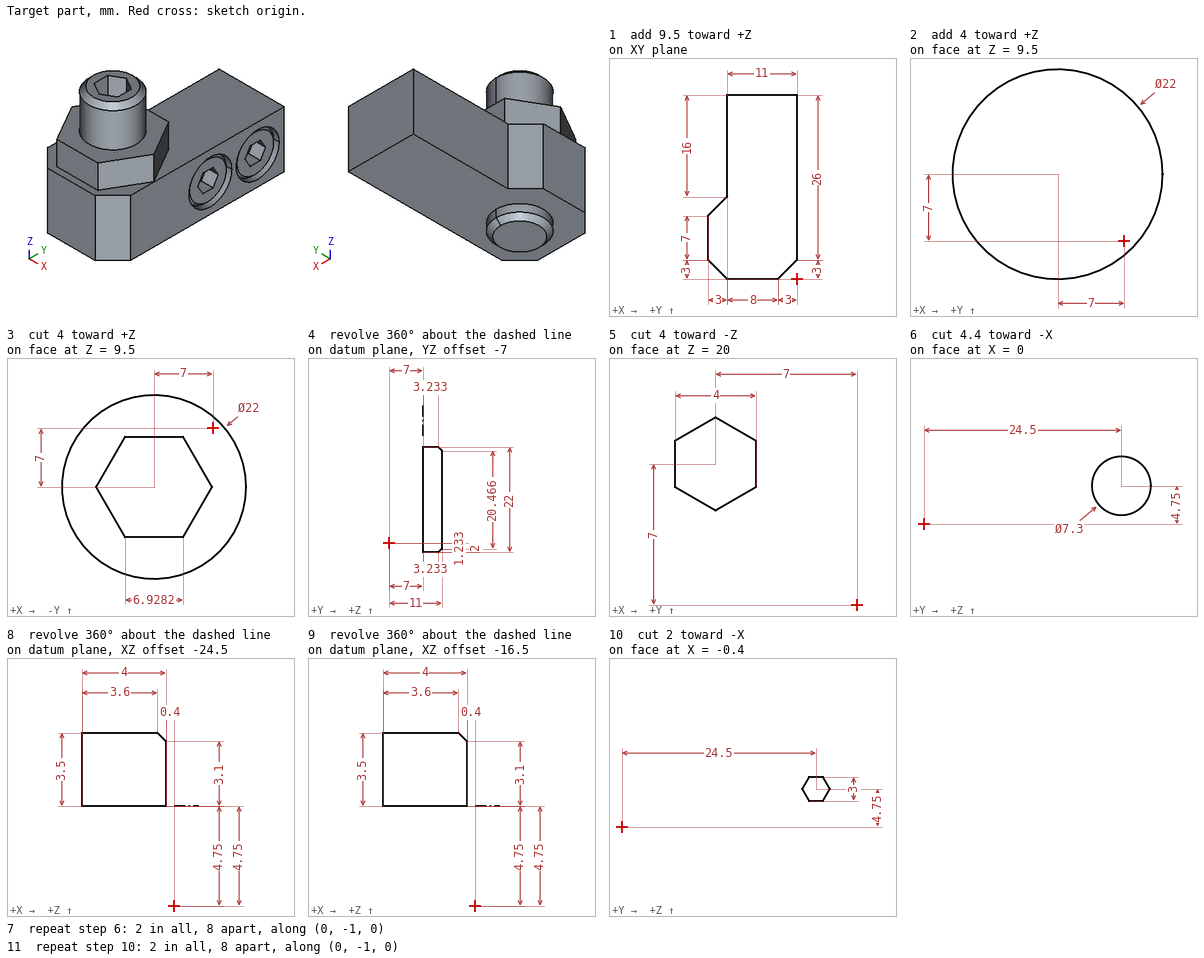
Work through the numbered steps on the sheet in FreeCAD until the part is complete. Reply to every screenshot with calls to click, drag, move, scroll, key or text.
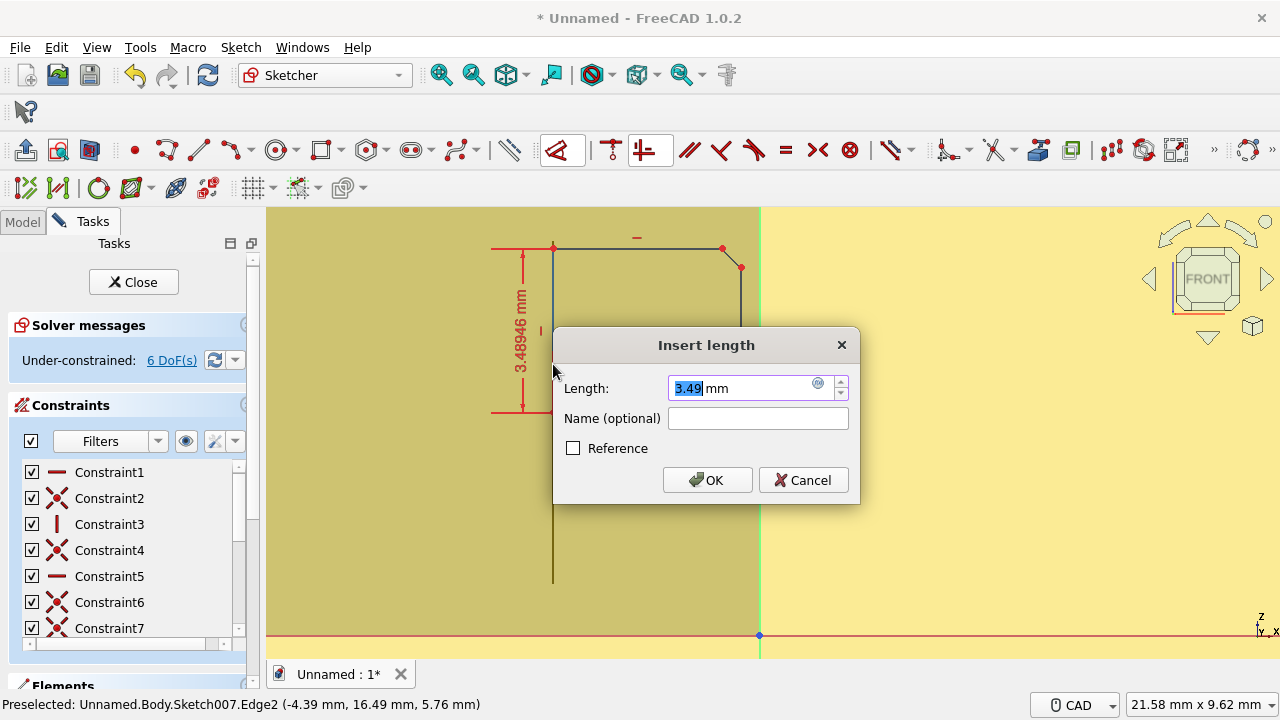
text(3.5)
key(Return)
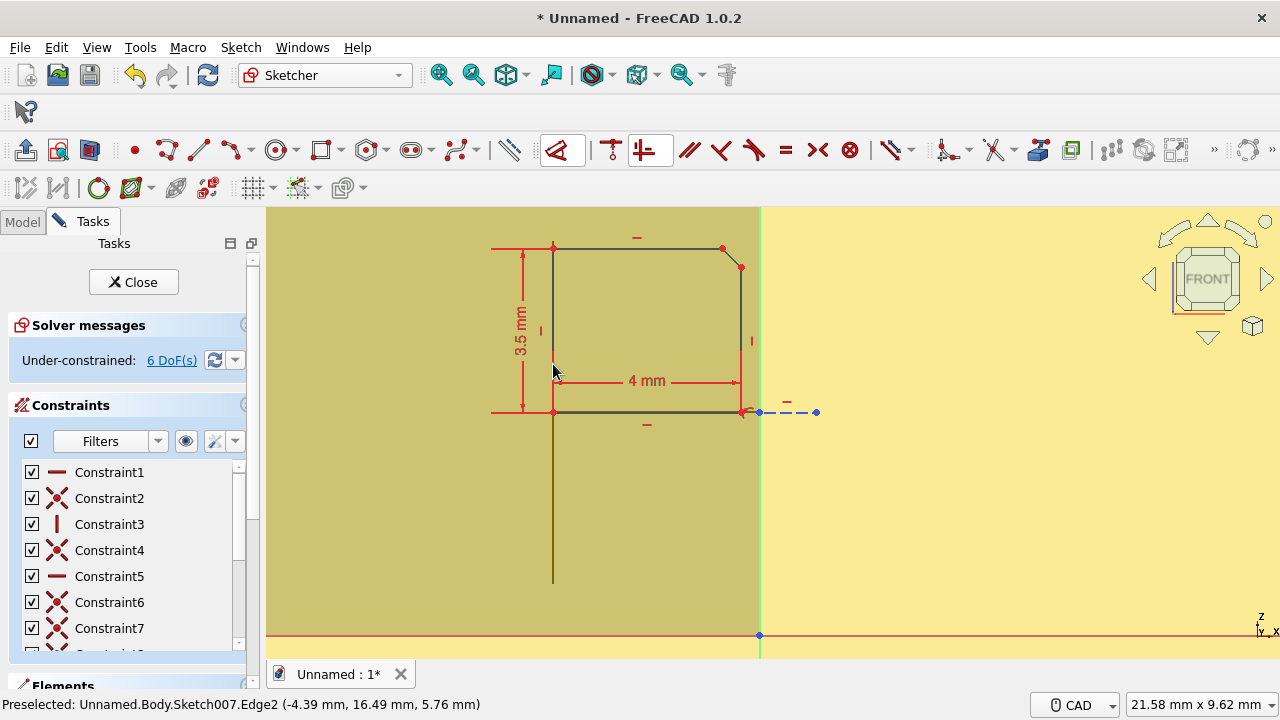
click(604, 249)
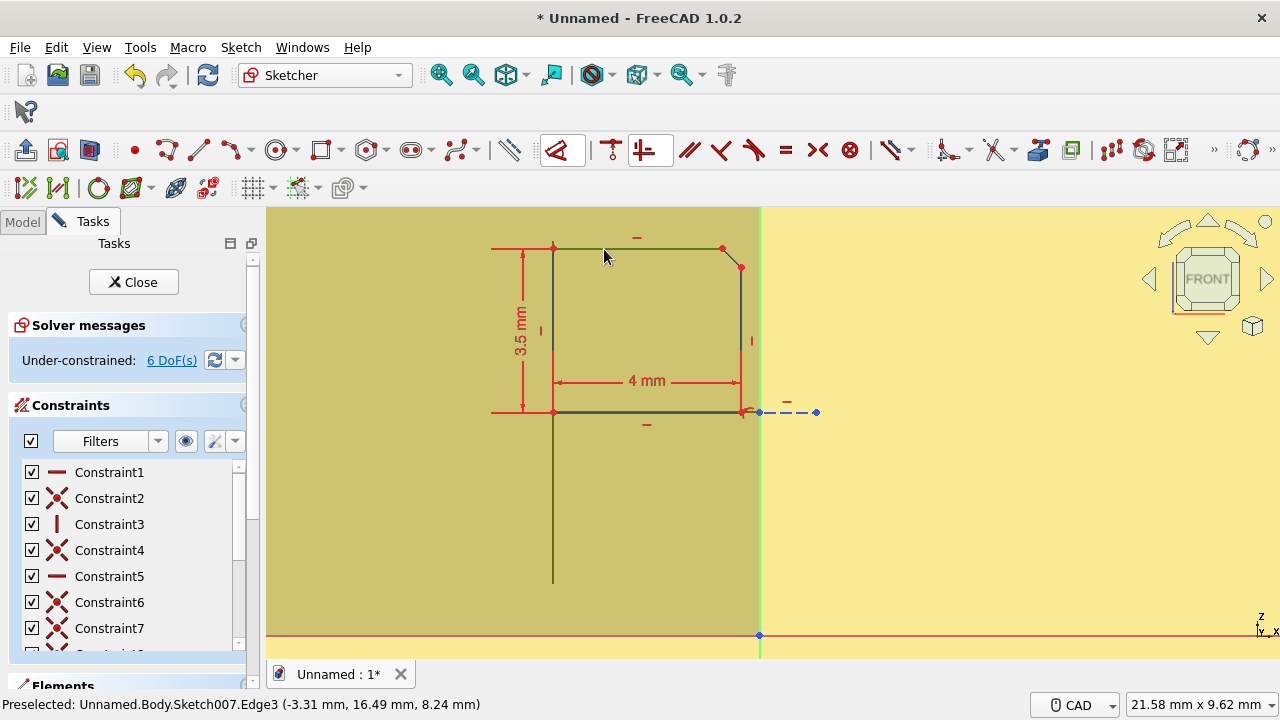
key(l)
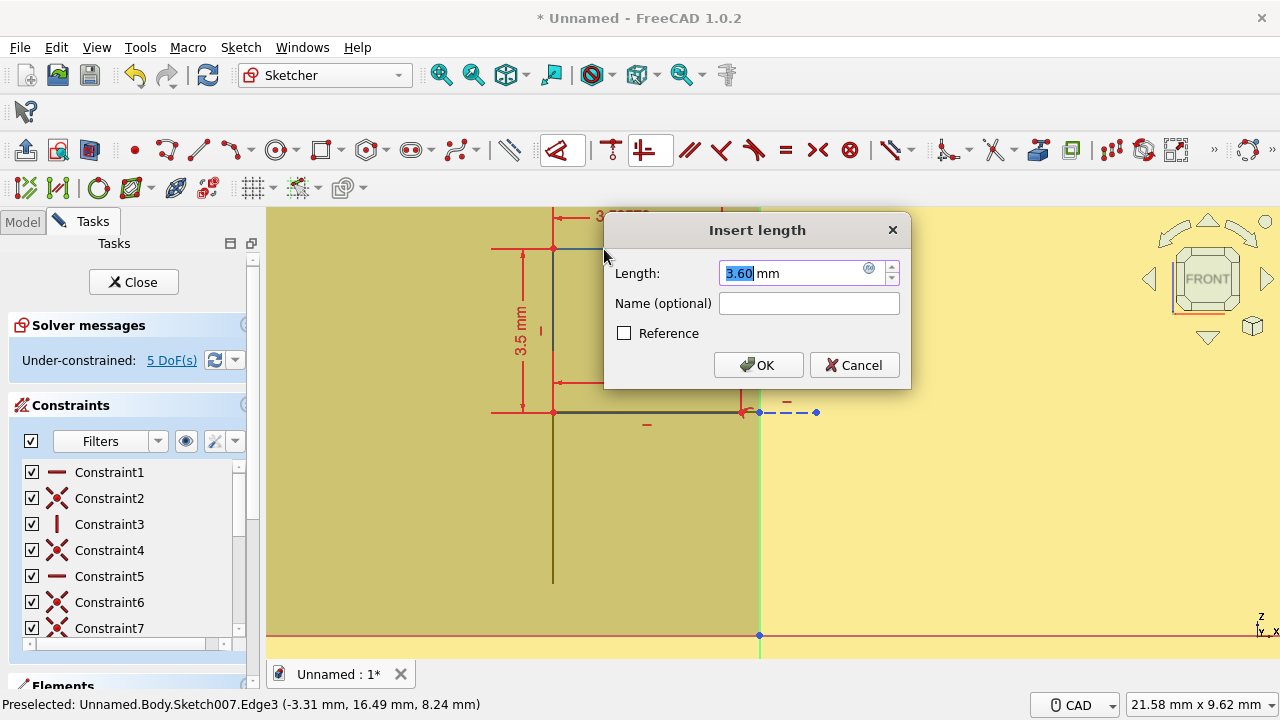
text(3.6)
key(Return)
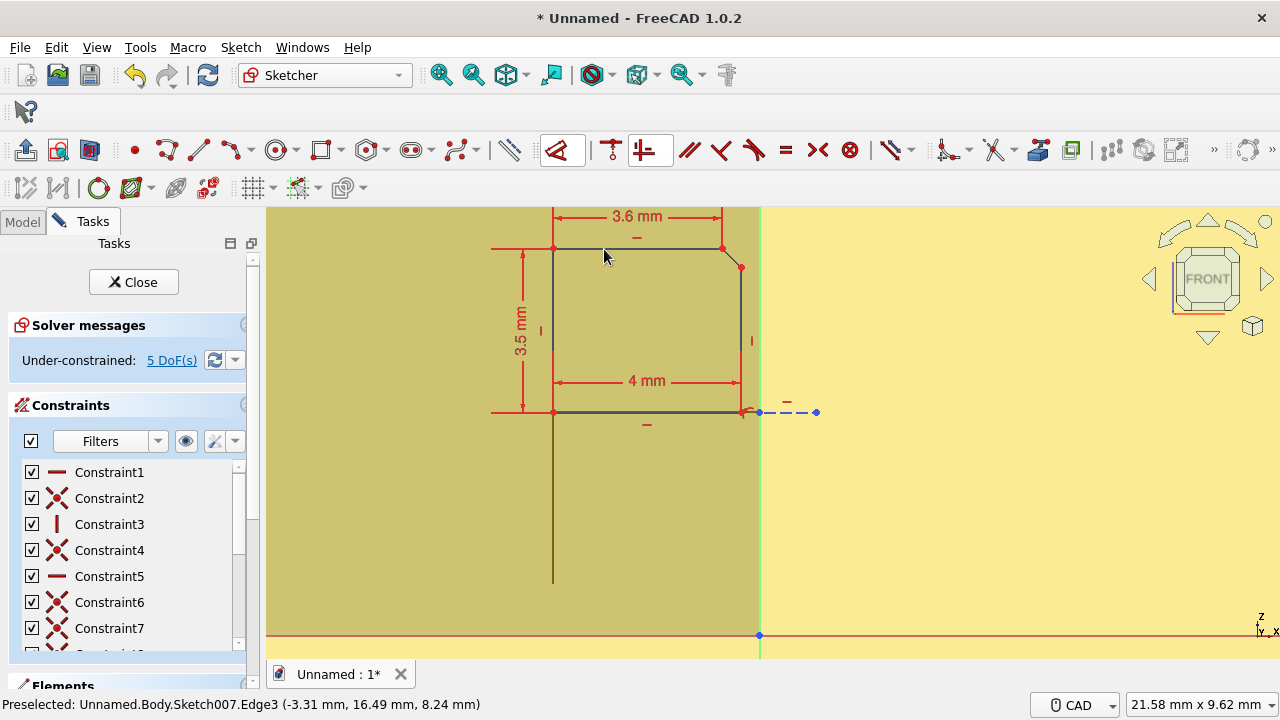
click(741, 312)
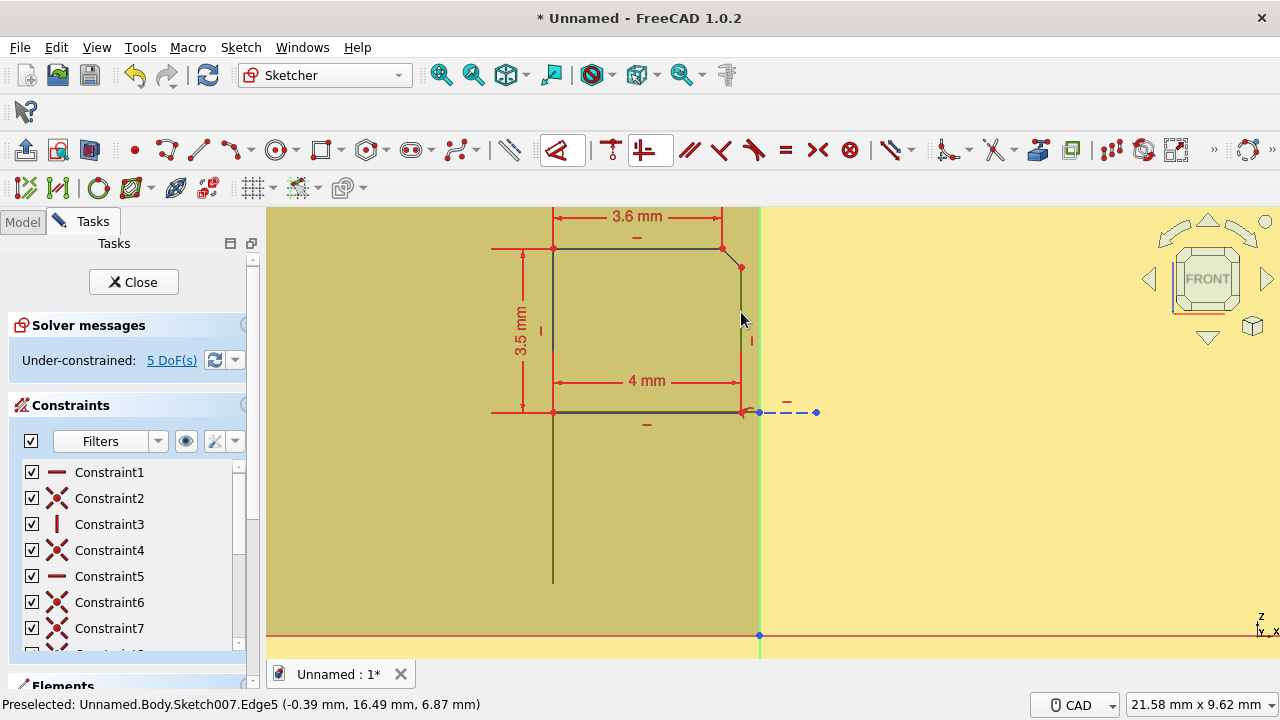
click(580, 150)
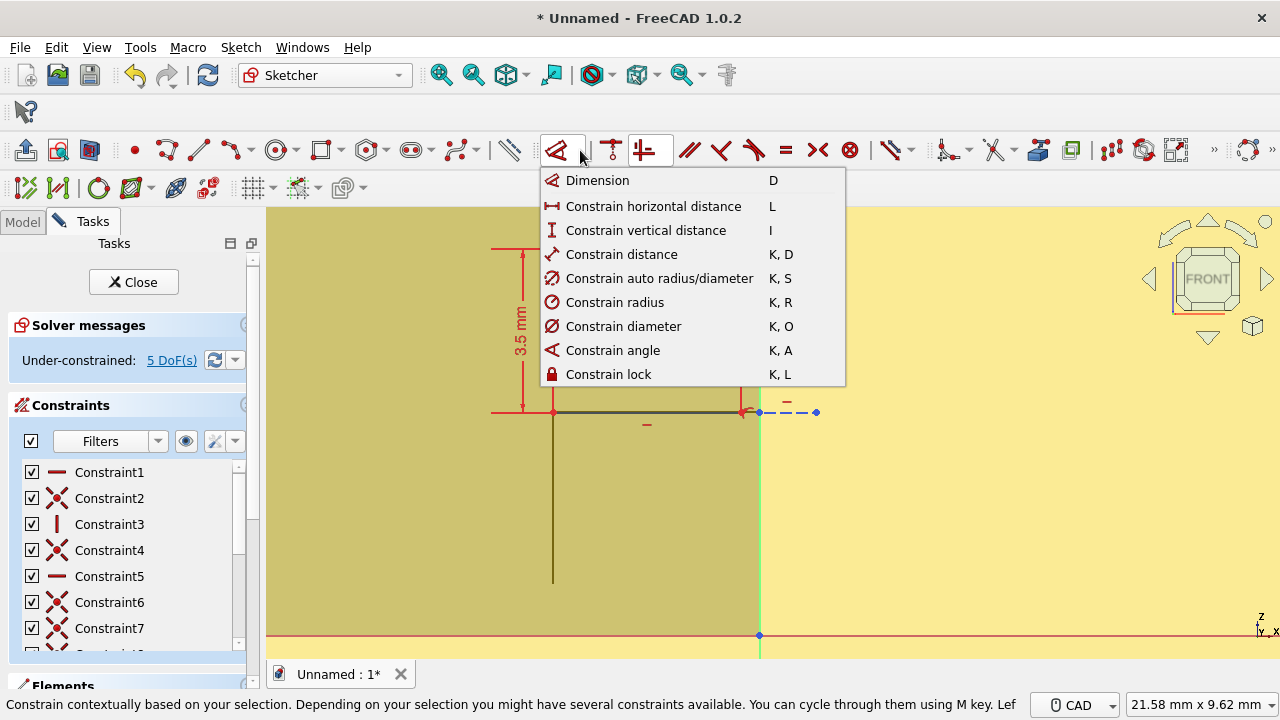
click(693, 230)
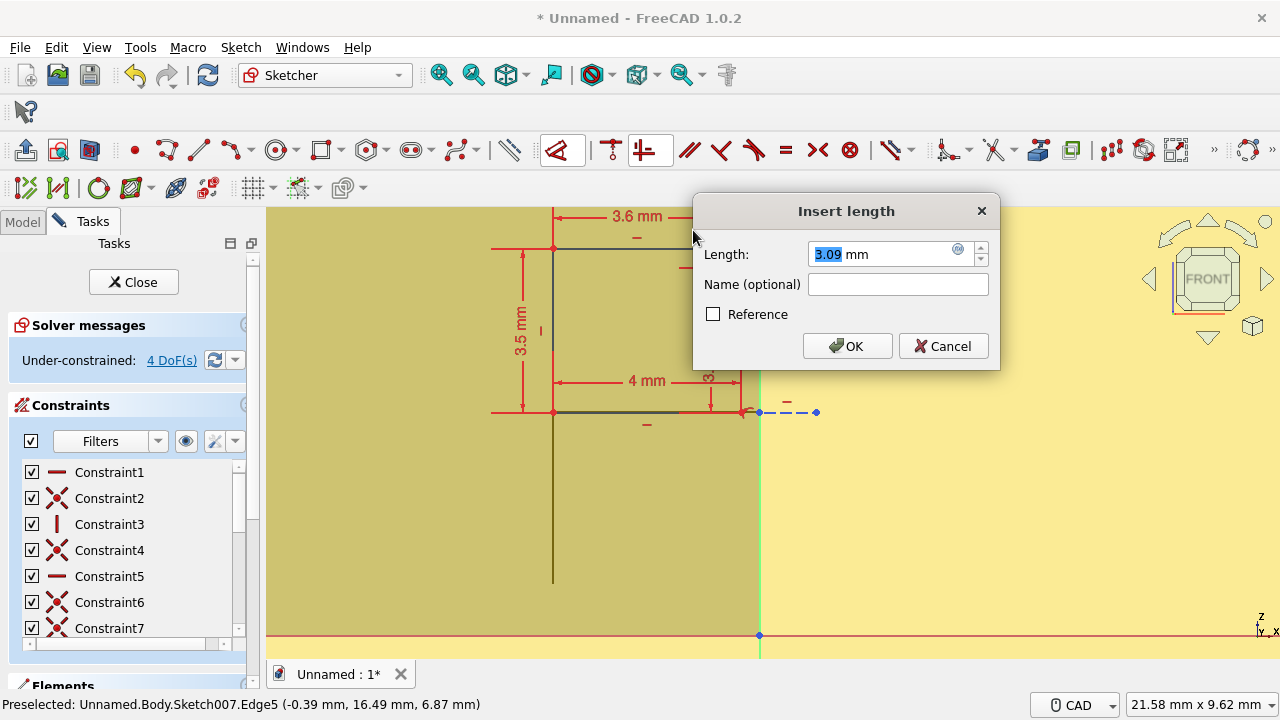
text(3.1)
key(Return)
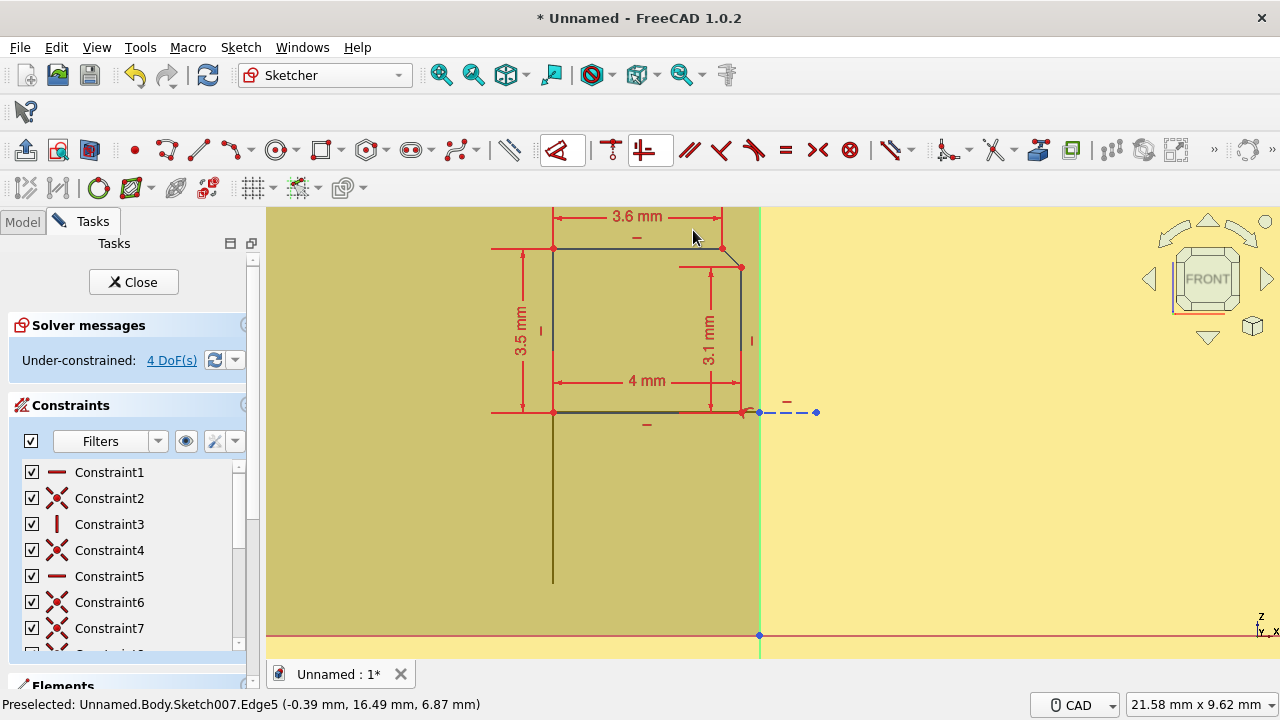
scroll(741, 413, up, 4)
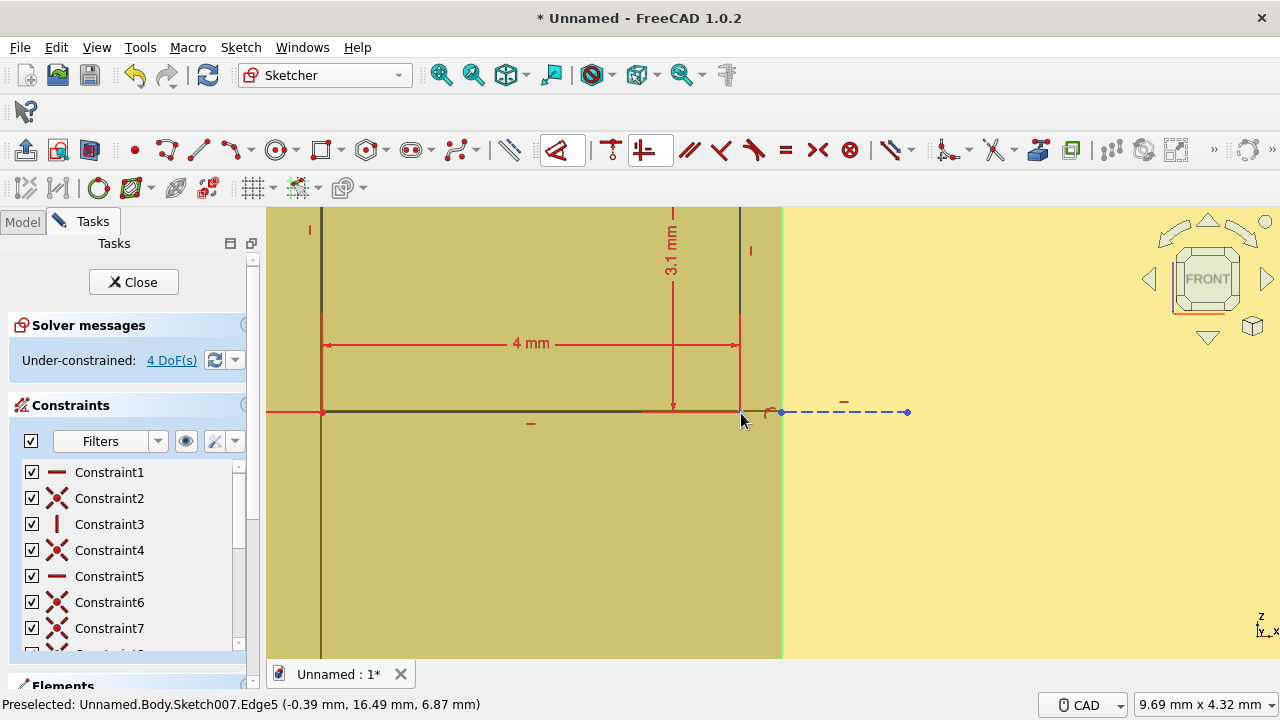
click(740, 412)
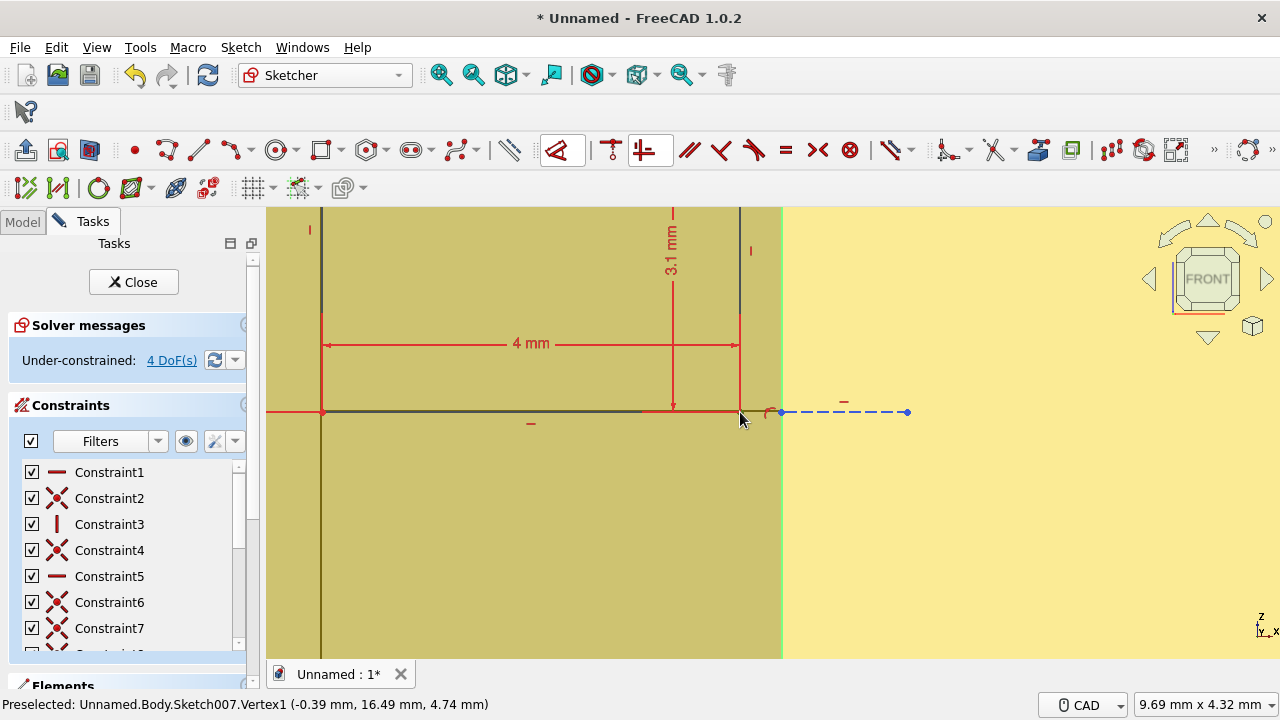
key(l)